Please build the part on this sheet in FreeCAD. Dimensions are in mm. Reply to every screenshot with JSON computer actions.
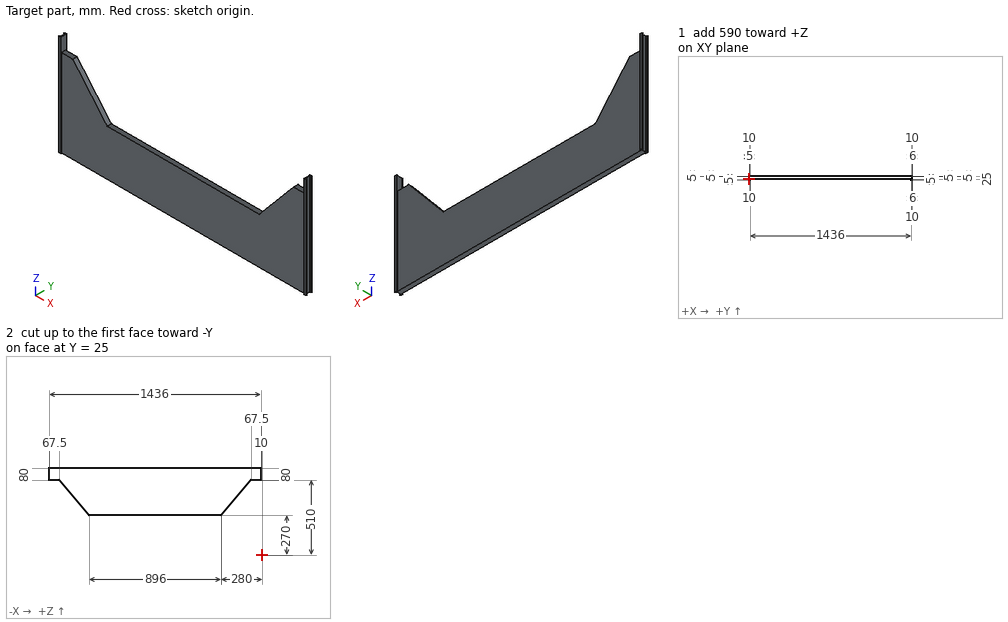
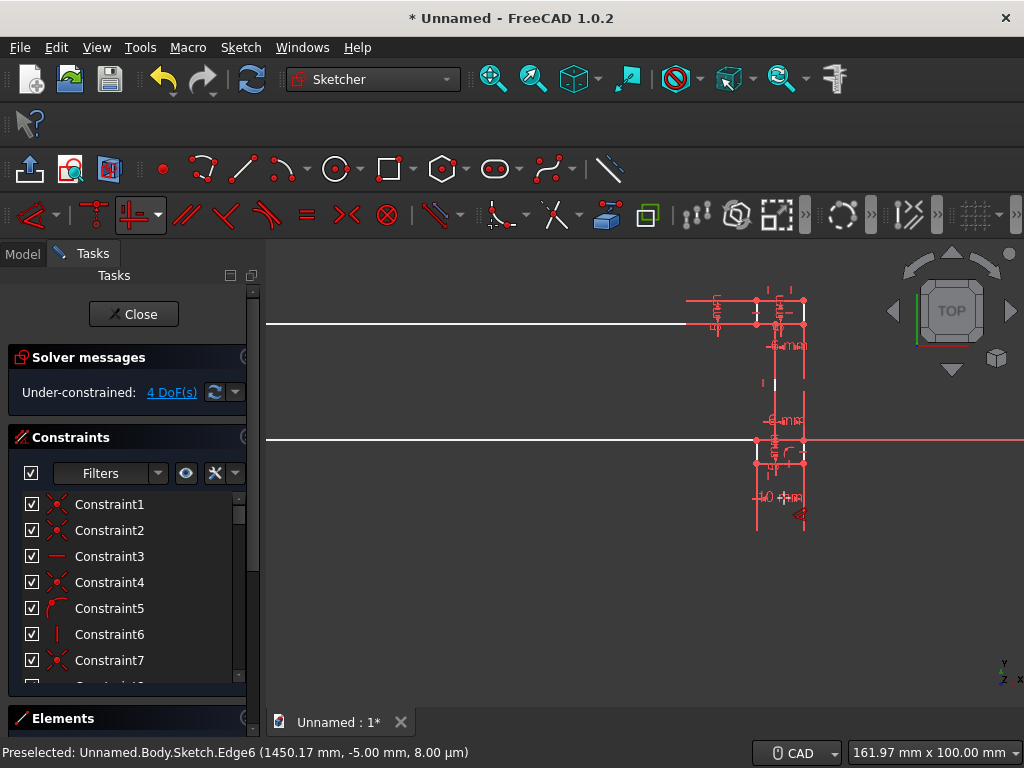
{"action": "left_click", "coordinate": [775, 405]}
{"action": "left_click", "coordinate": [809, 382]}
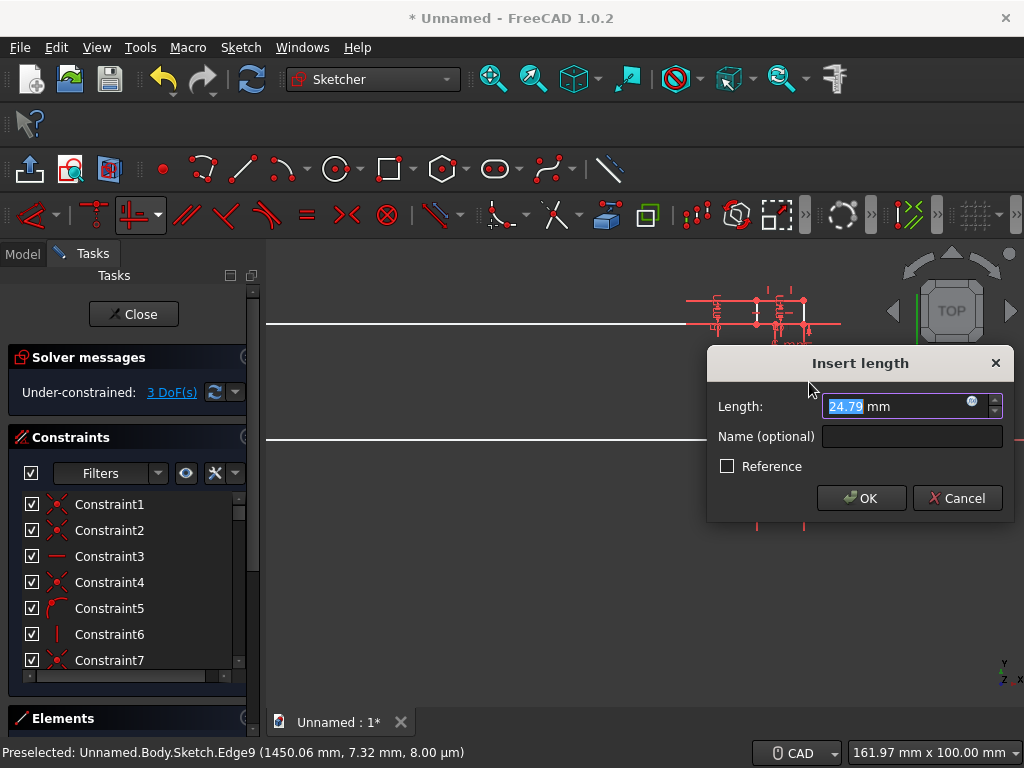
{"action": "type", "text": "25"}
{"action": "key", "text": "Return"}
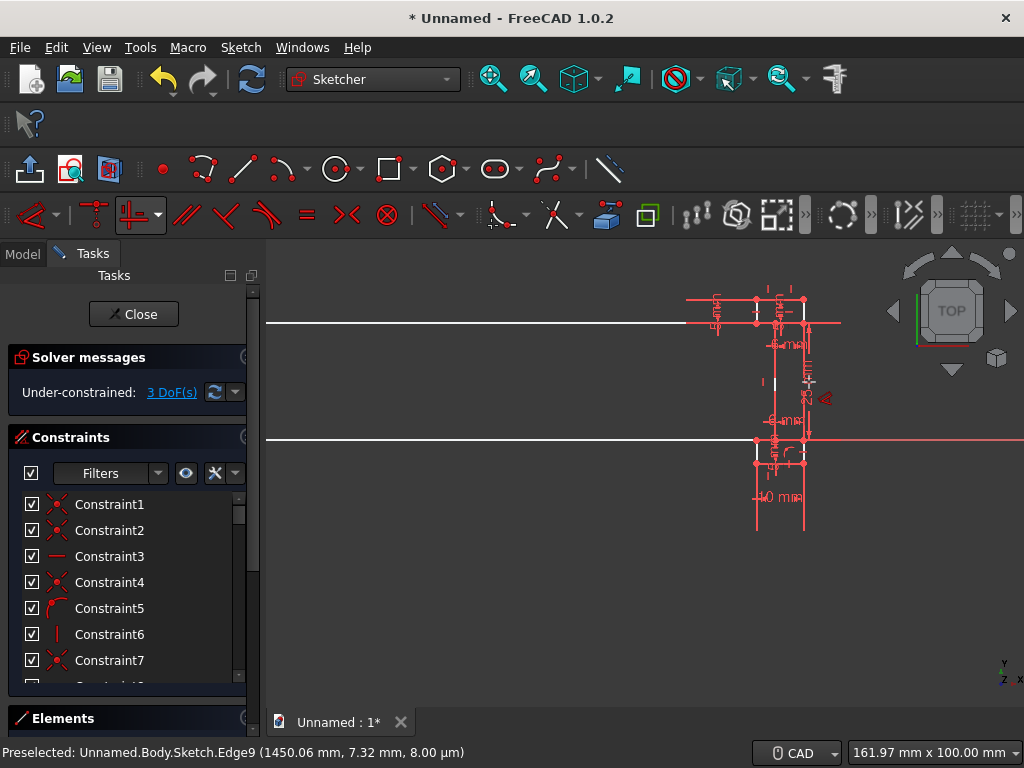
{"action": "left_click", "coordinate": [790, 300]}
{"action": "left_click", "coordinate": [791, 334]}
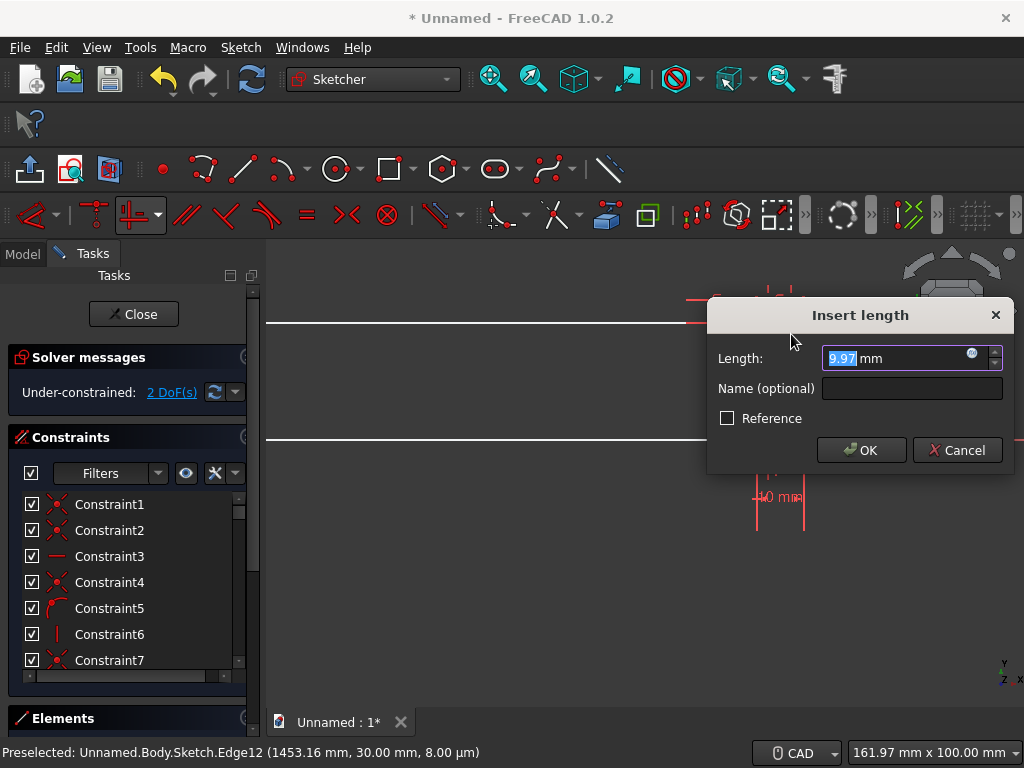
{"action": "type", "text": "10"}
{"action": "key", "text": "Return"}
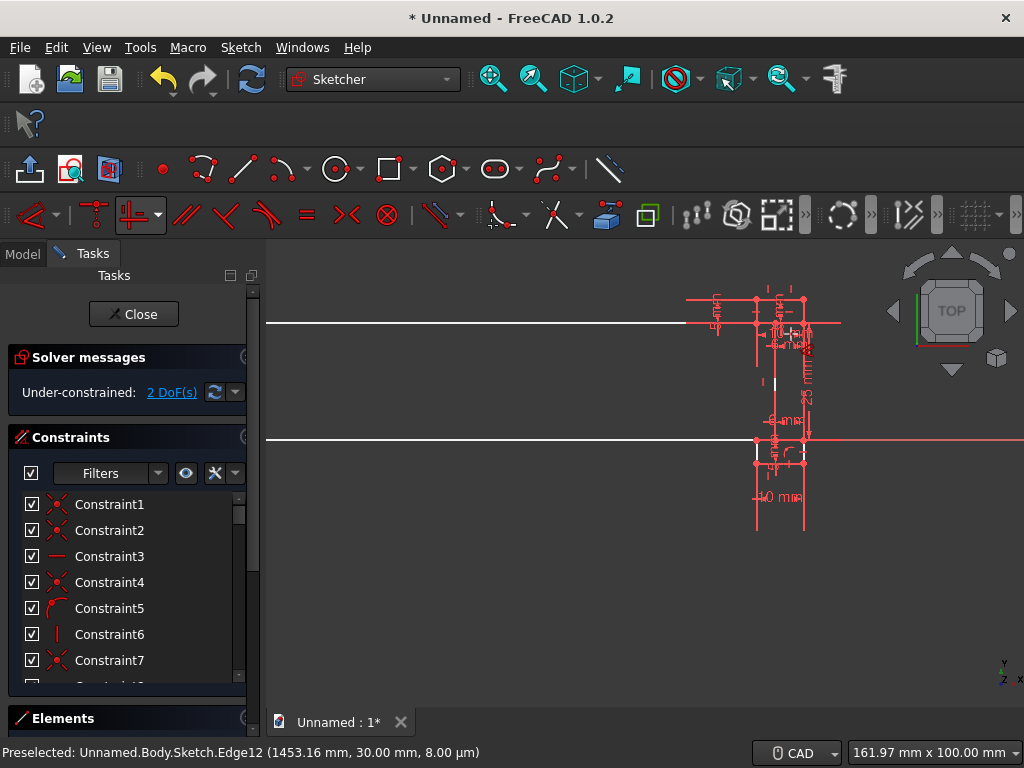
{"action": "scroll", "coordinate": [782, 479], "scroll_direction": "down", "scroll_amount": 14}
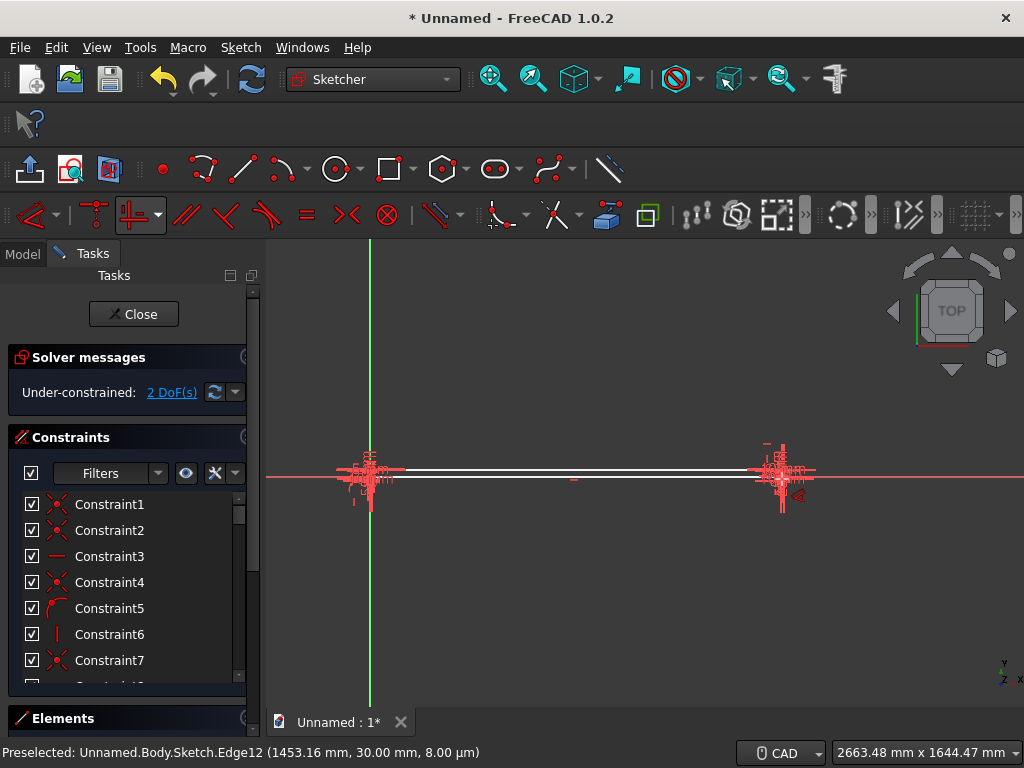
{"action": "scroll", "coordinate": [372, 469], "scroll_direction": "up", "scroll_amount": 14}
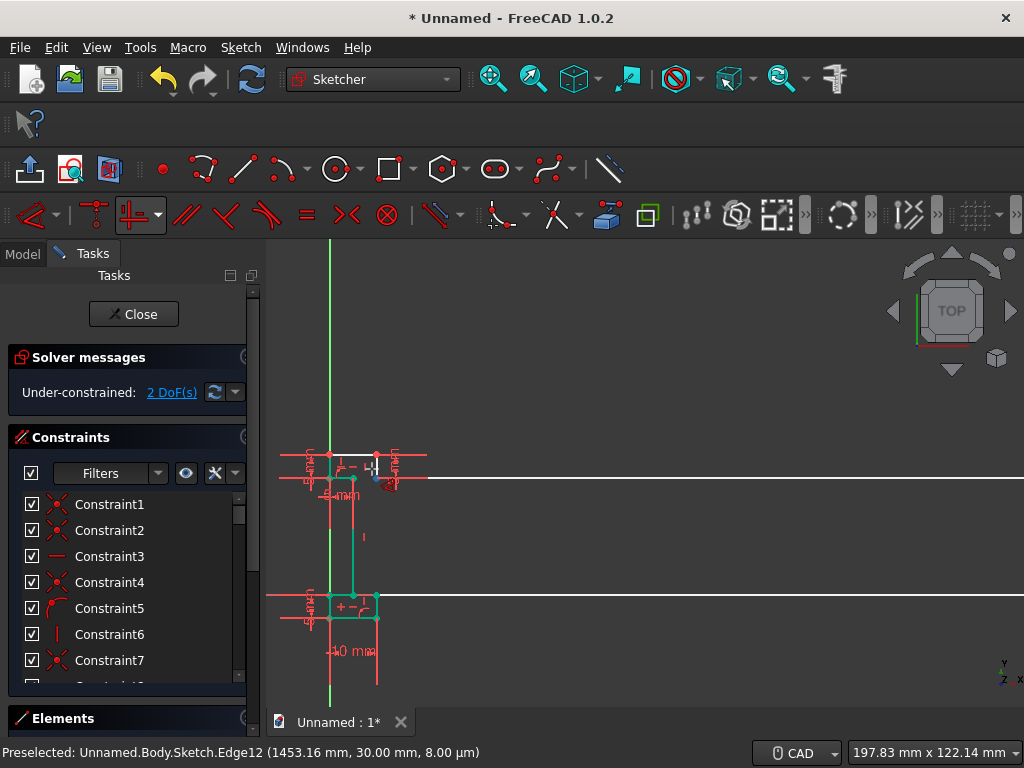
{"action": "left_click", "coordinate": [363, 455]}
{"action": "left_click", "coordinate": [353, 421]}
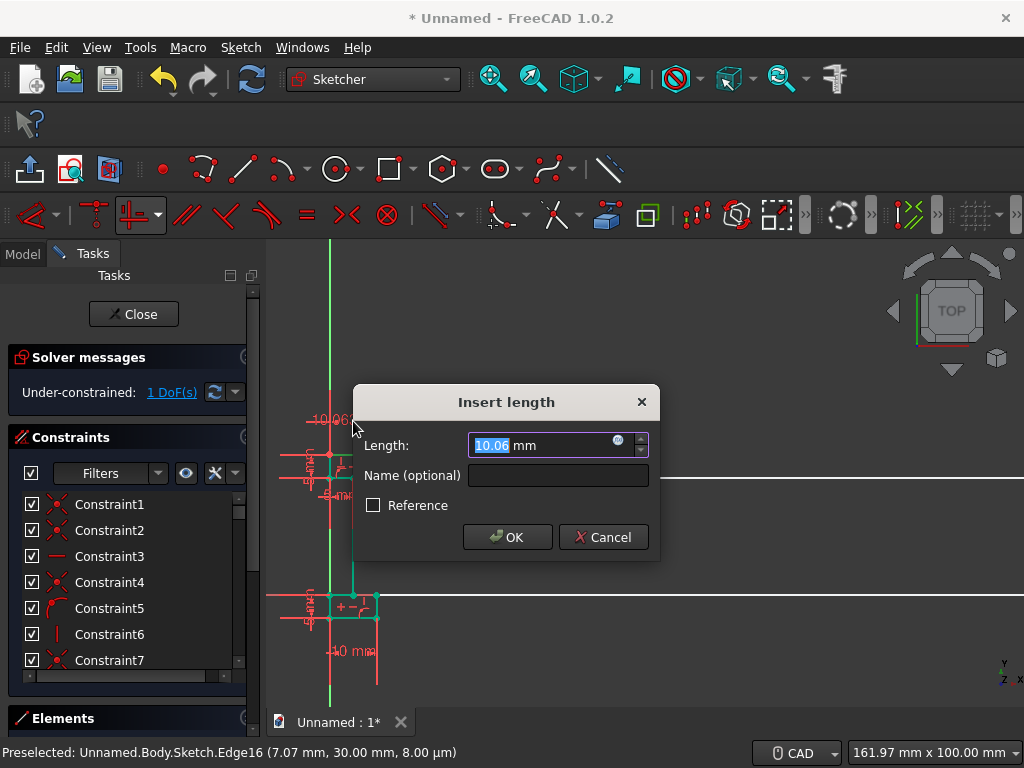
{"action": "type", "text": "10"}
{"action": "key", "text": "Return"}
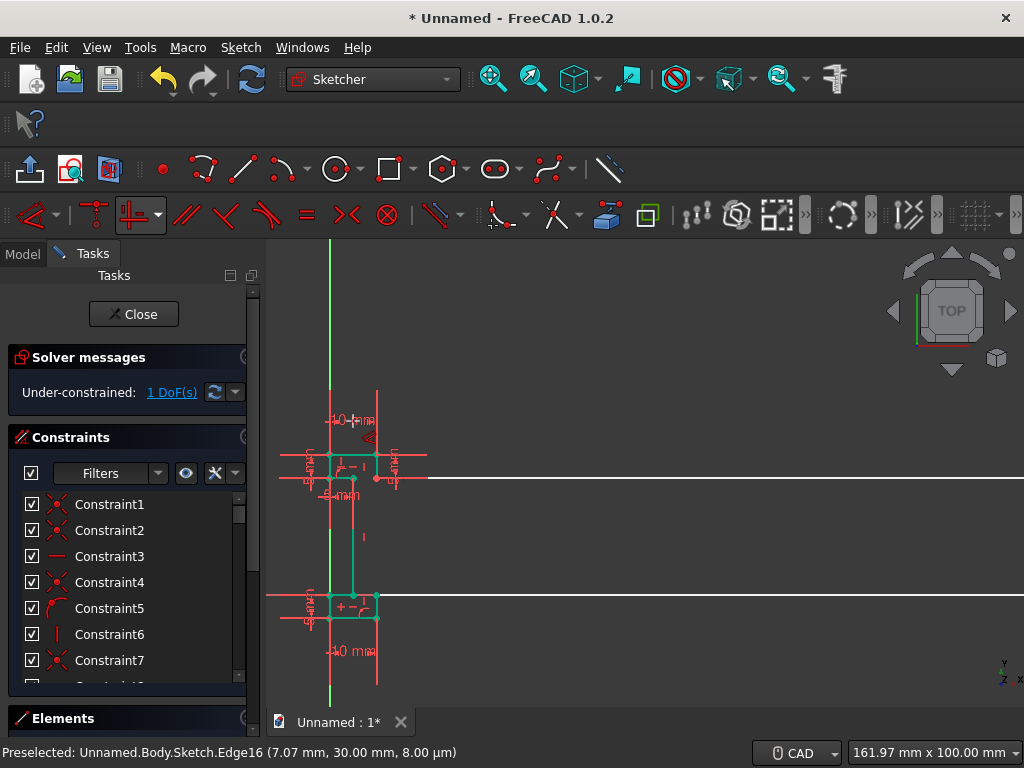
{"action": "scroll", "coordinate": [372, 469], "scroll_direction": "down", "scroll_amount": 14}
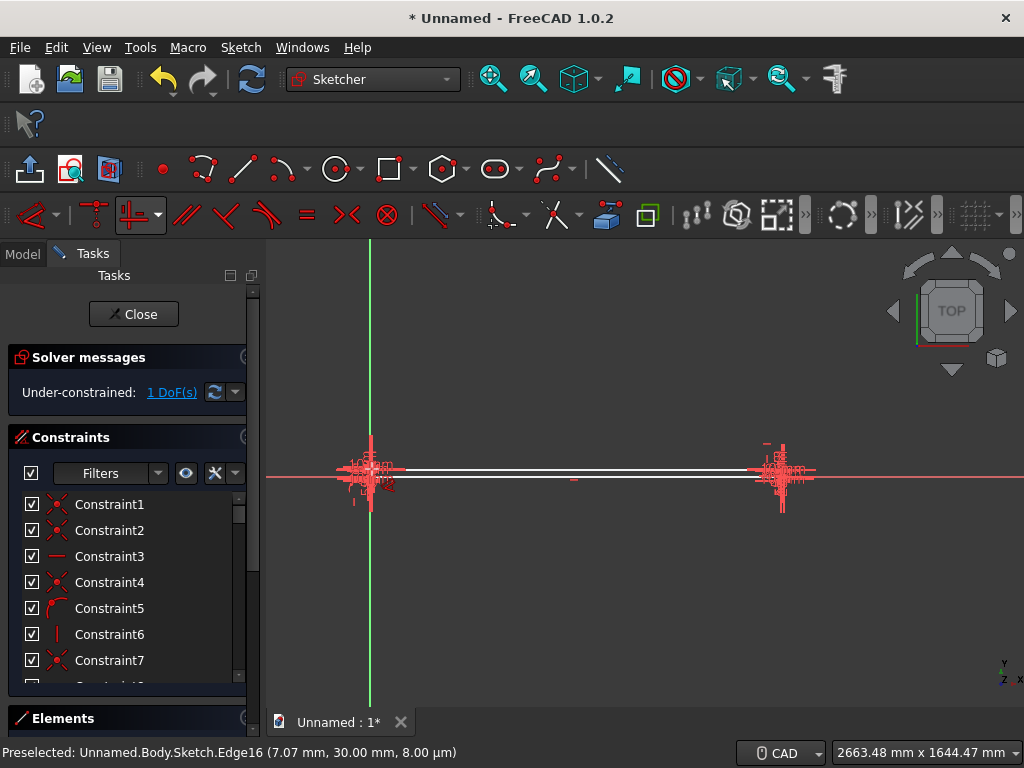
{"action": "scroll", "coordinate": [495, 477], "scroll_direction": "up", "scroll_amount": 4}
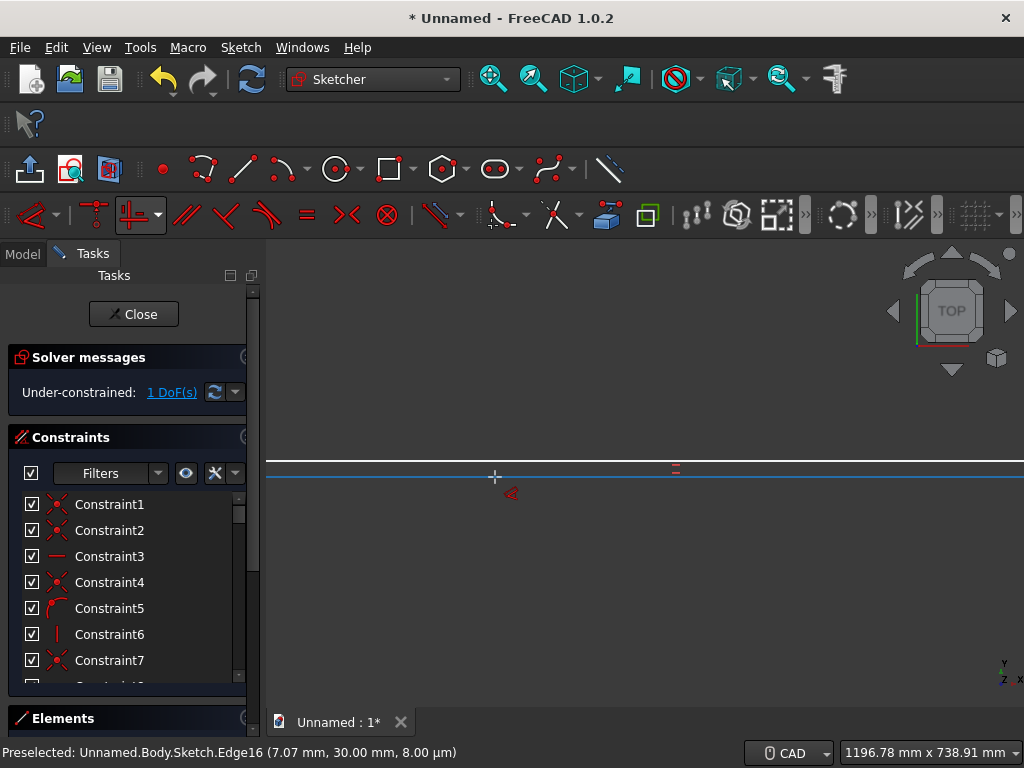
{"action": "left_click", "coordinate": [495, 477]}
{"action": "left_click", "coordinate": [576, 511]}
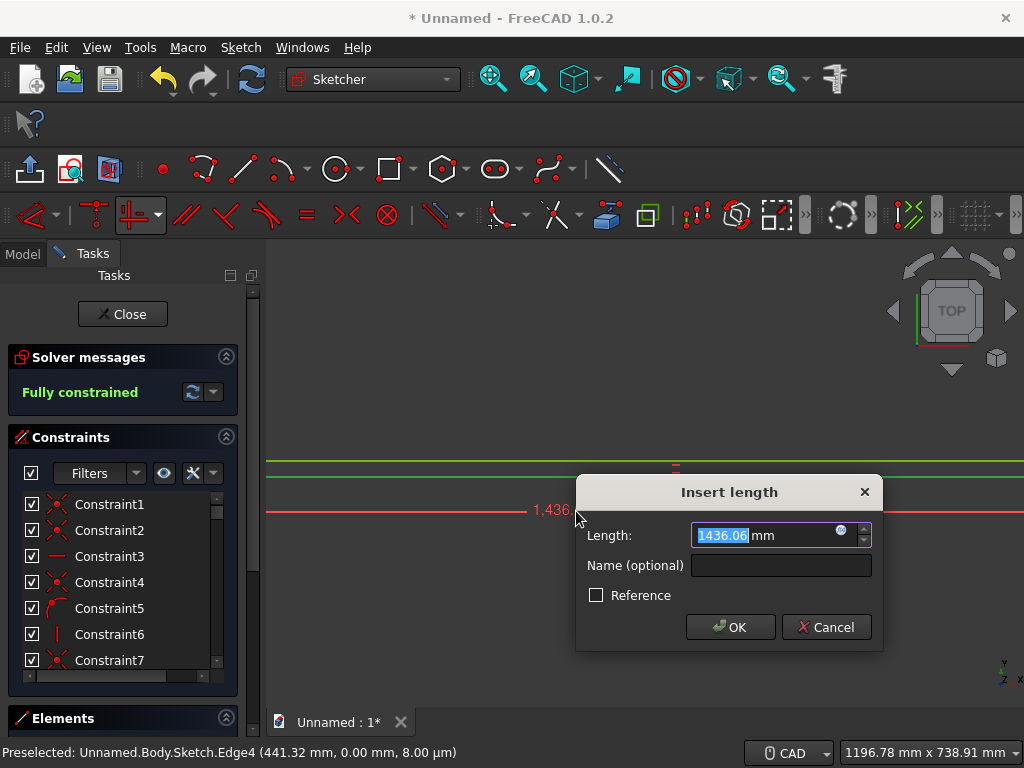
{"action": "type", "text": "1436"}
{"action": "key", "text": "Return"}
{"action": "key", "text": "Escape"}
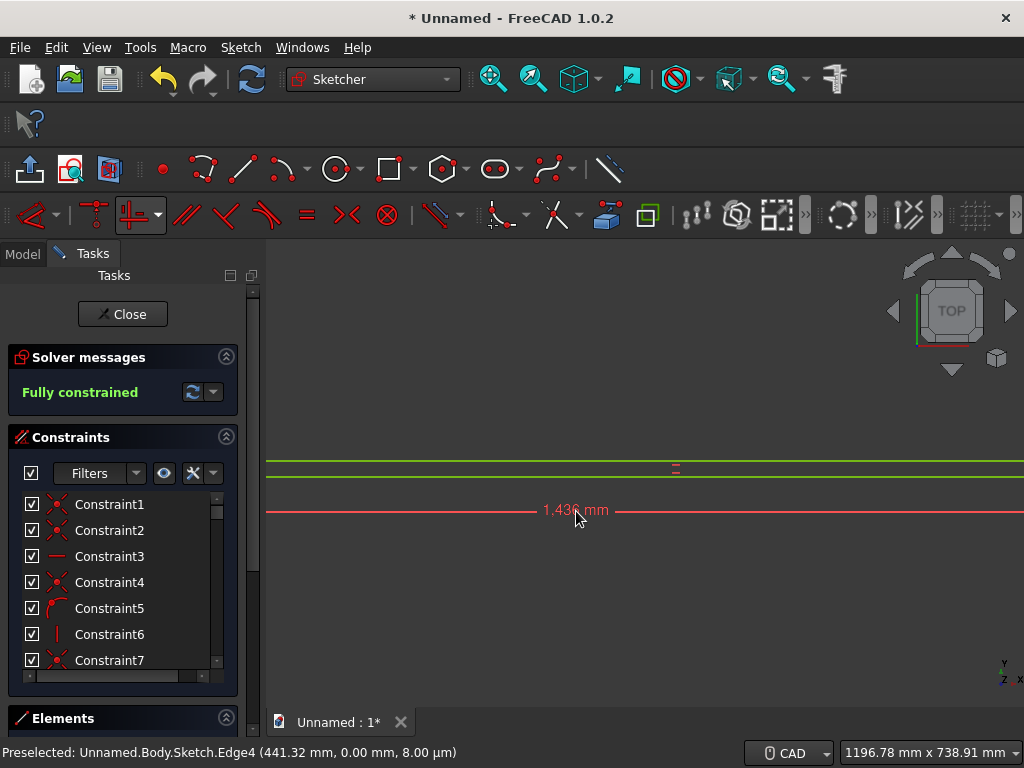
{"action": "left_click", "coordinate": [123, 314]}